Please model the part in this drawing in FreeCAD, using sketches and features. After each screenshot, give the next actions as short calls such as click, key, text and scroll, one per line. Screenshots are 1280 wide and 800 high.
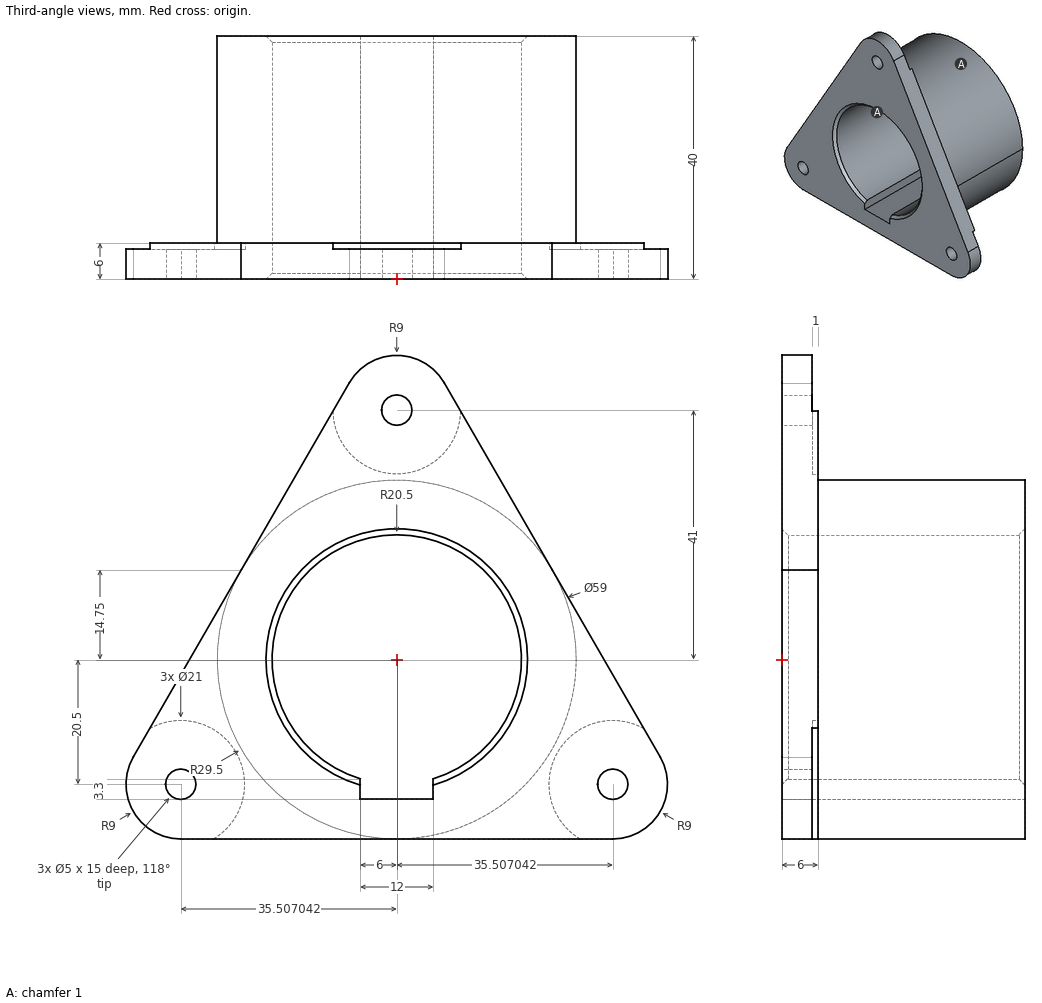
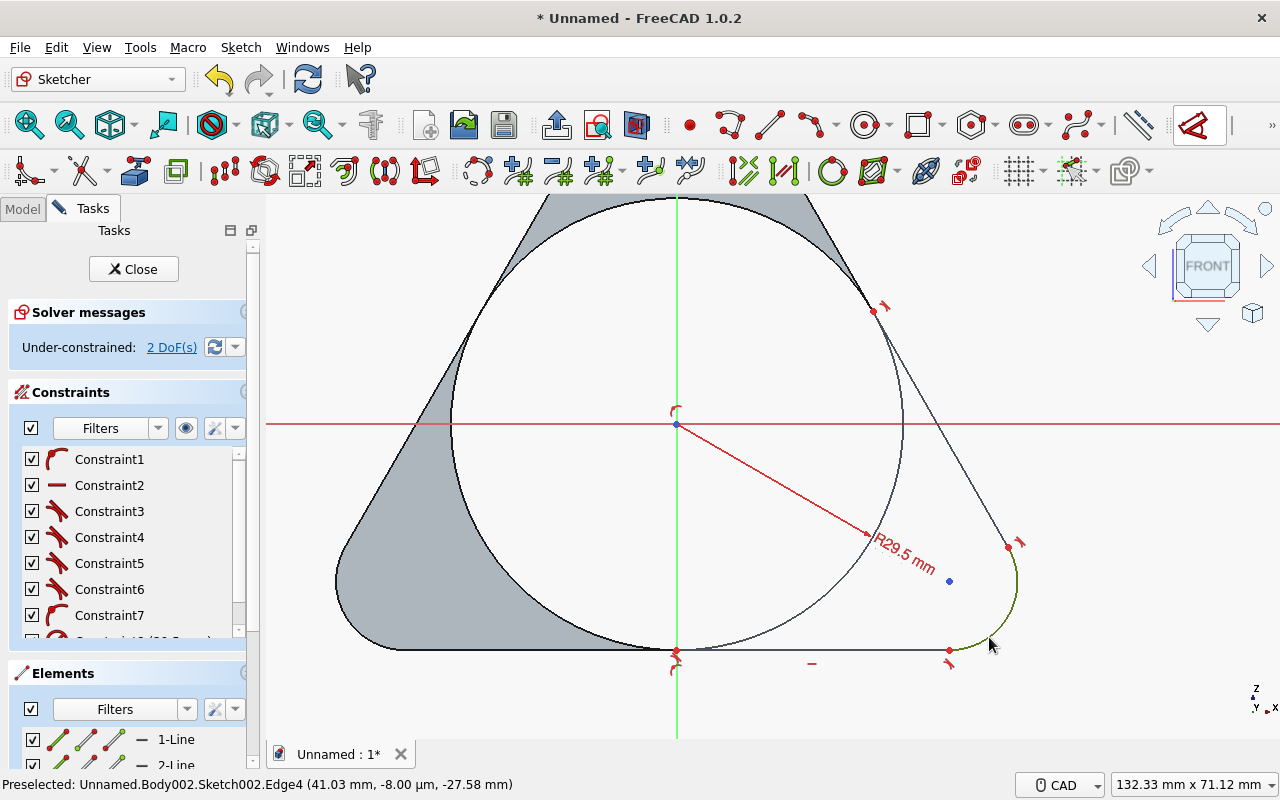
key(k)
key(r)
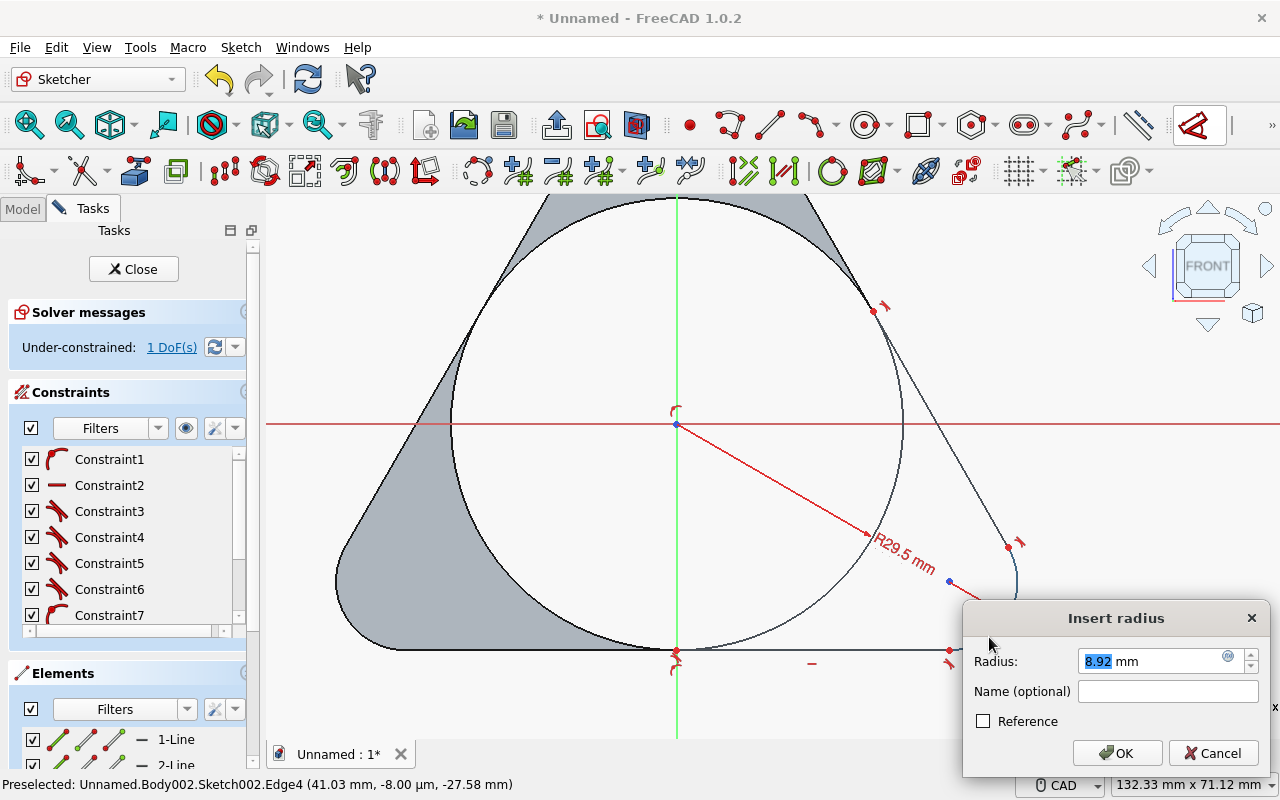
text(9)
key(Return)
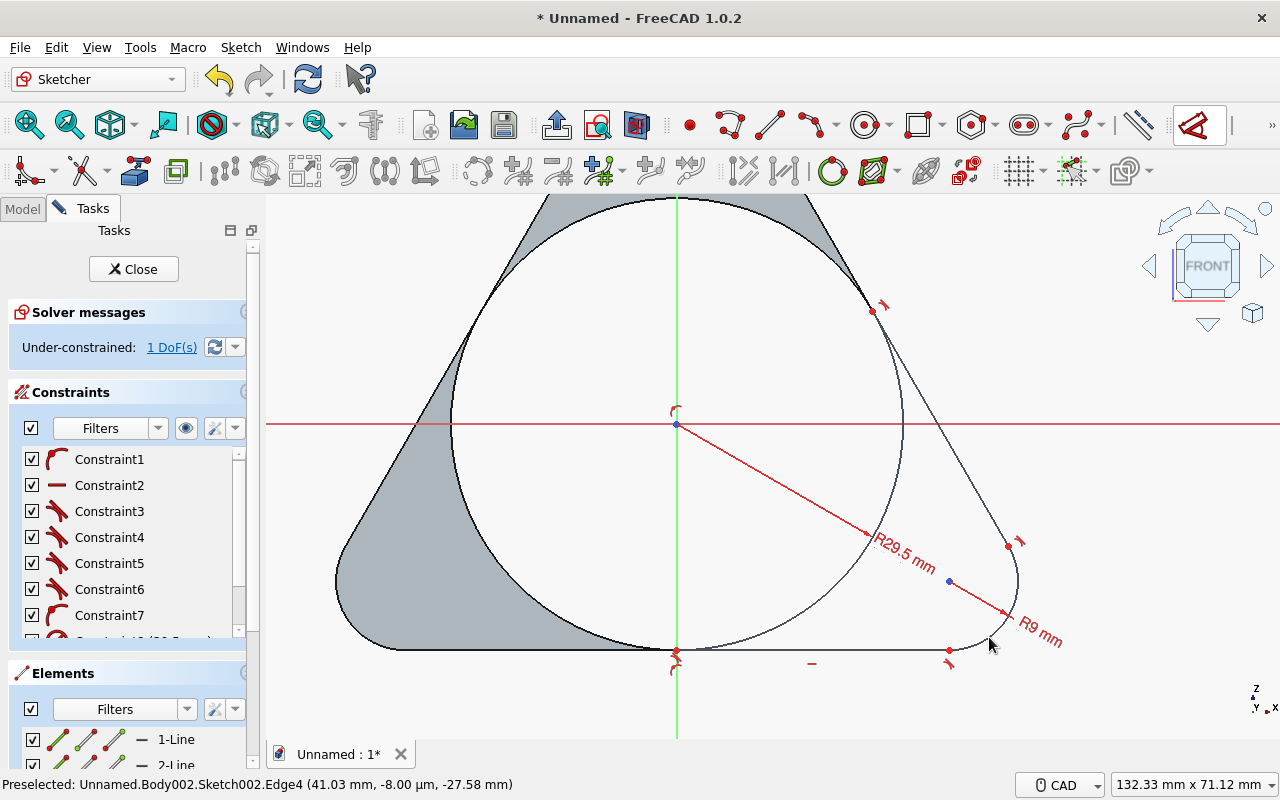
click(873, 311)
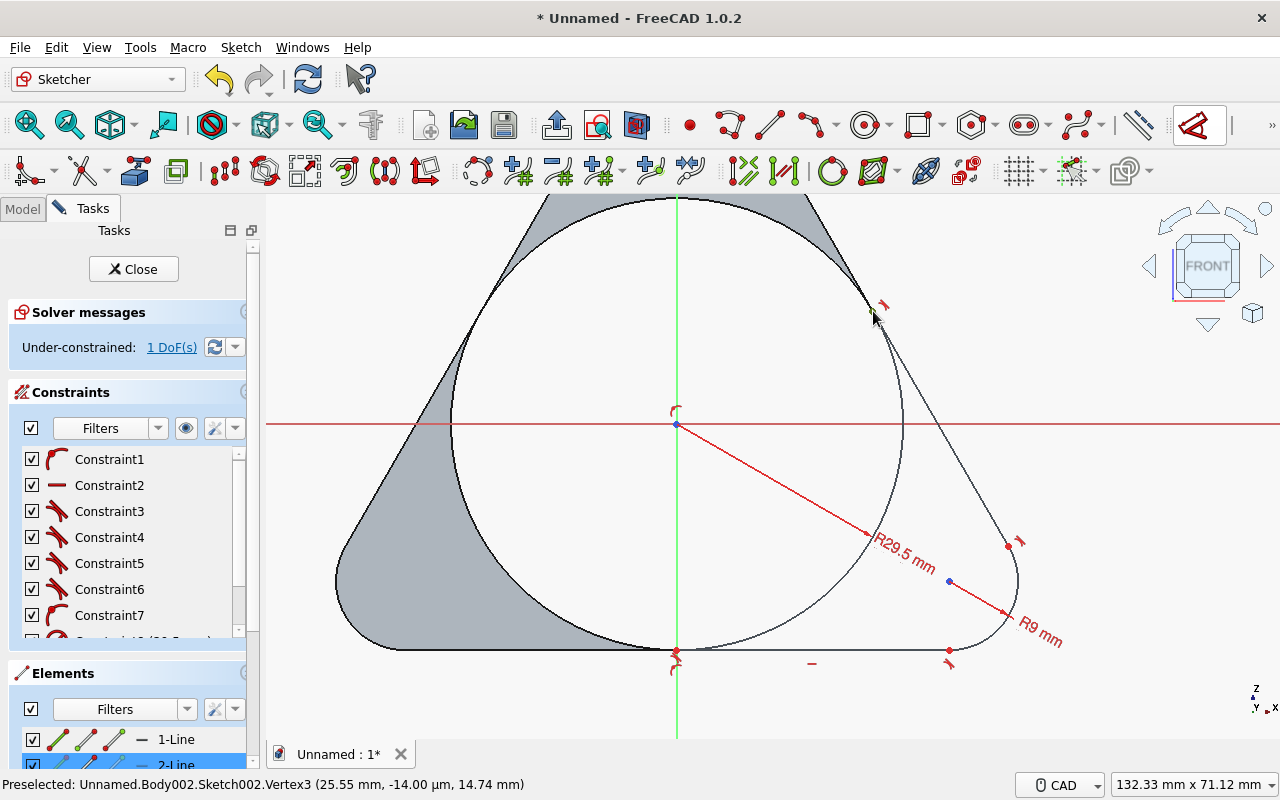
click(1220, 126)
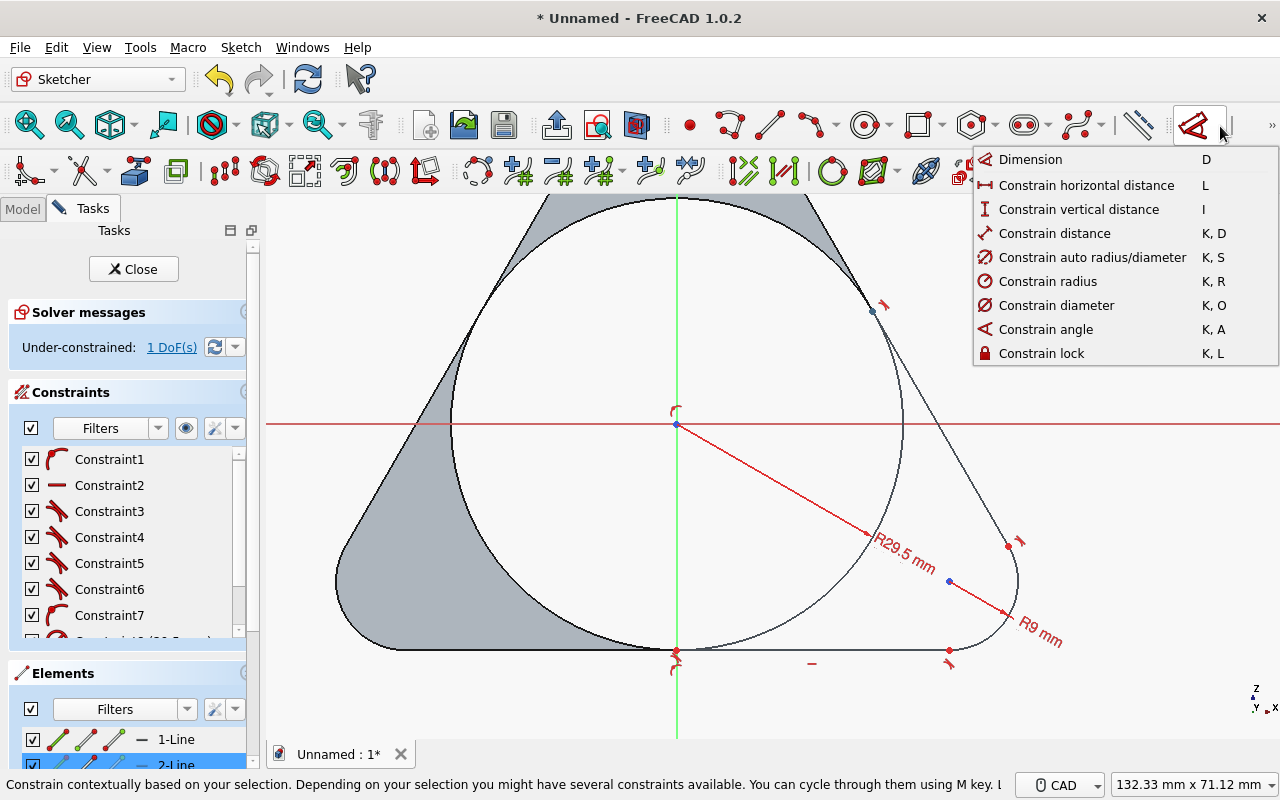
click(1126, 209)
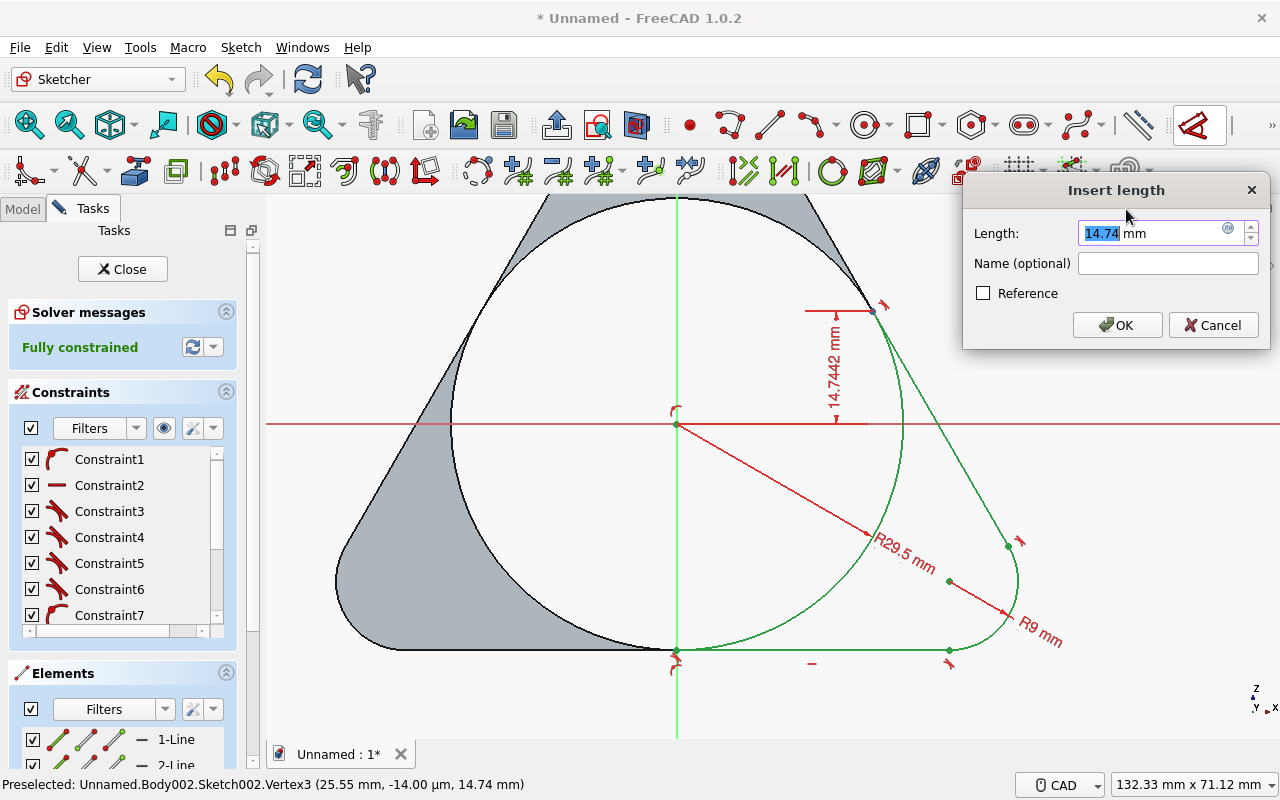
text(14.75)
key(Return)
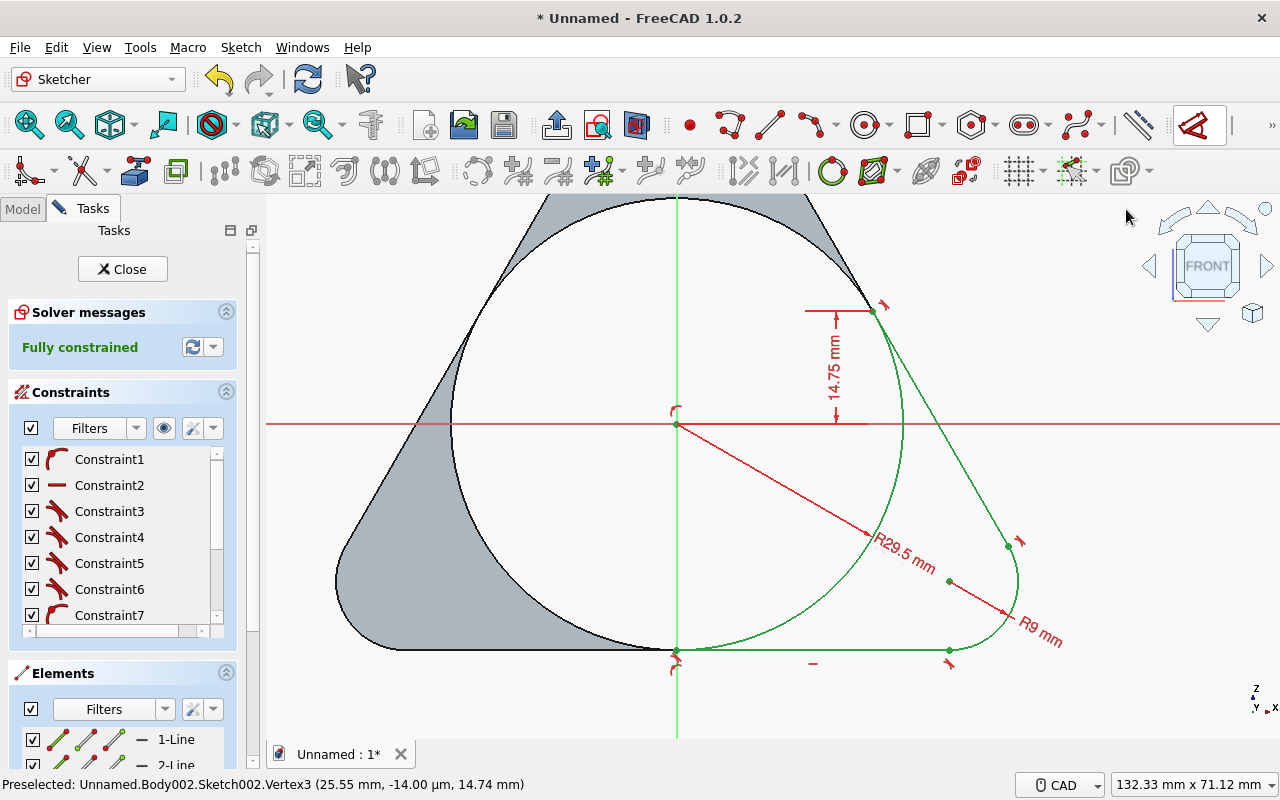
click(123, 269)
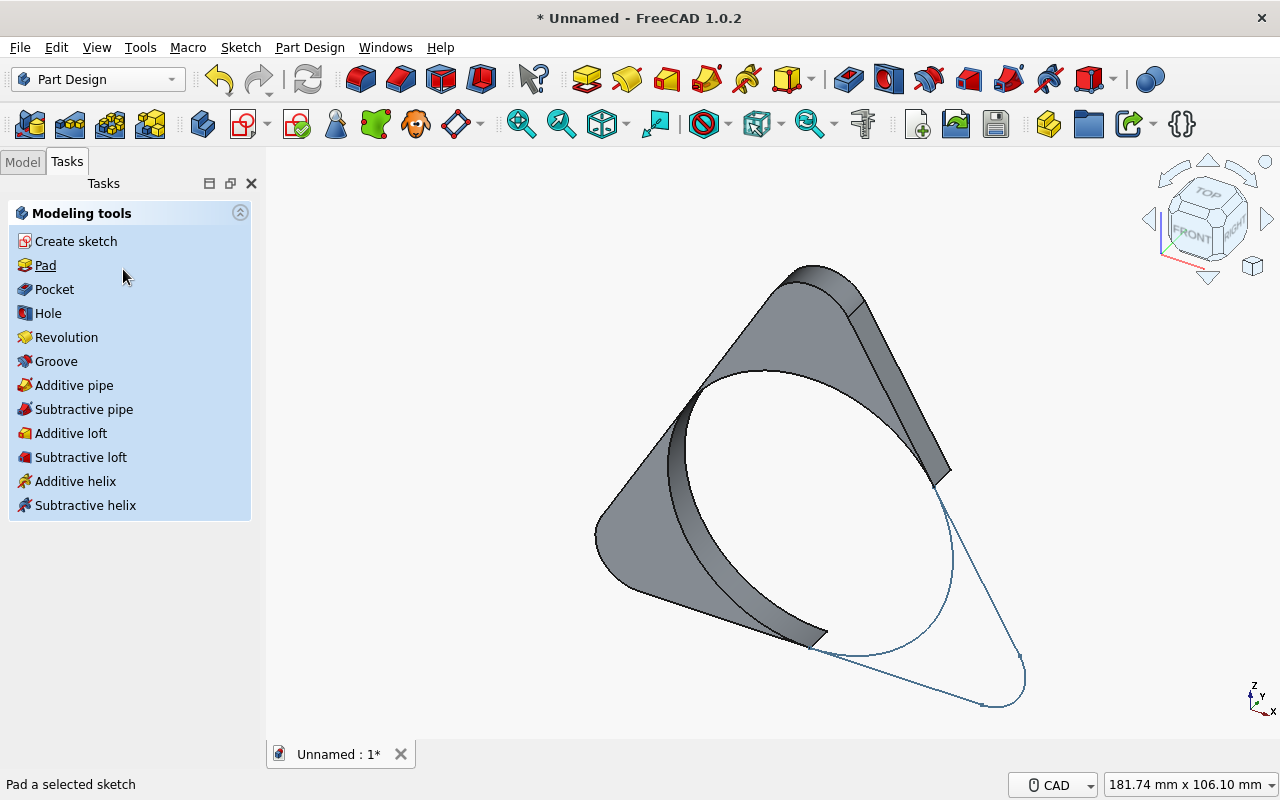
click(588, 80)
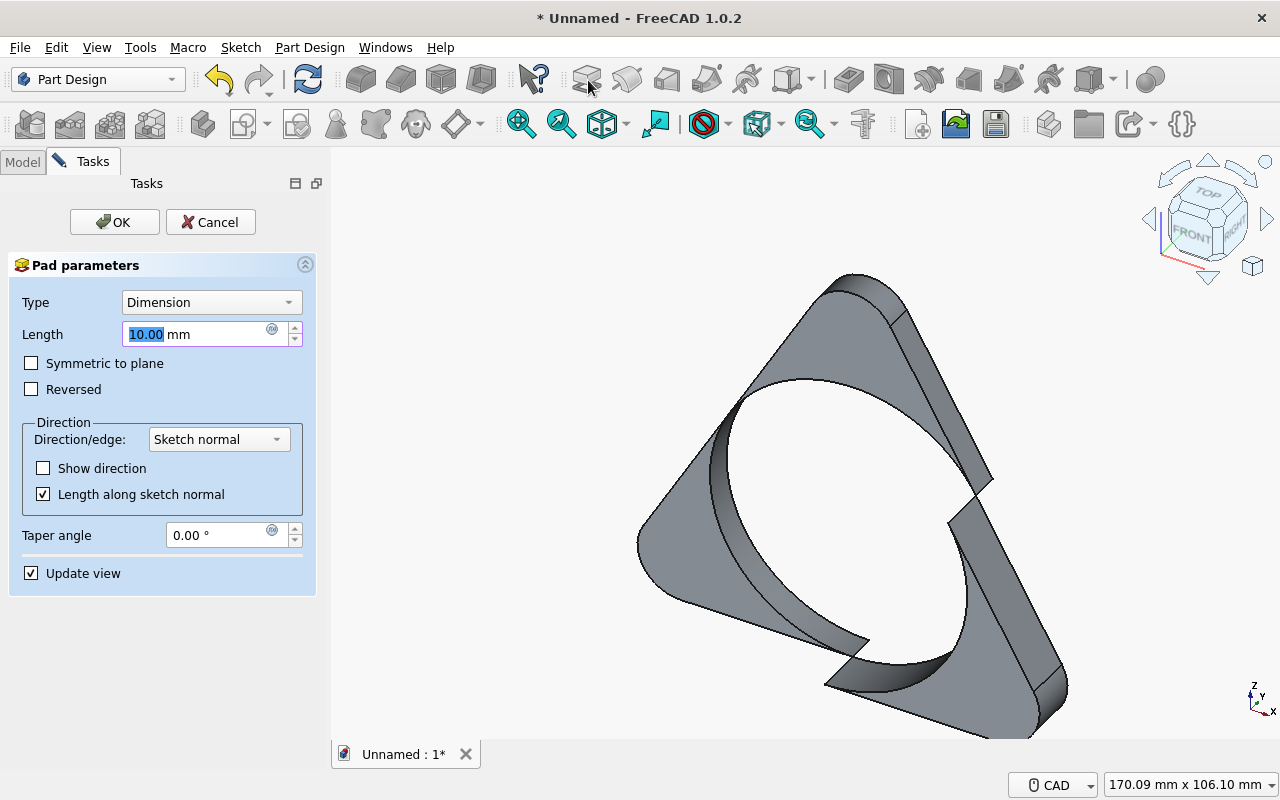
text(6)
key(Tab)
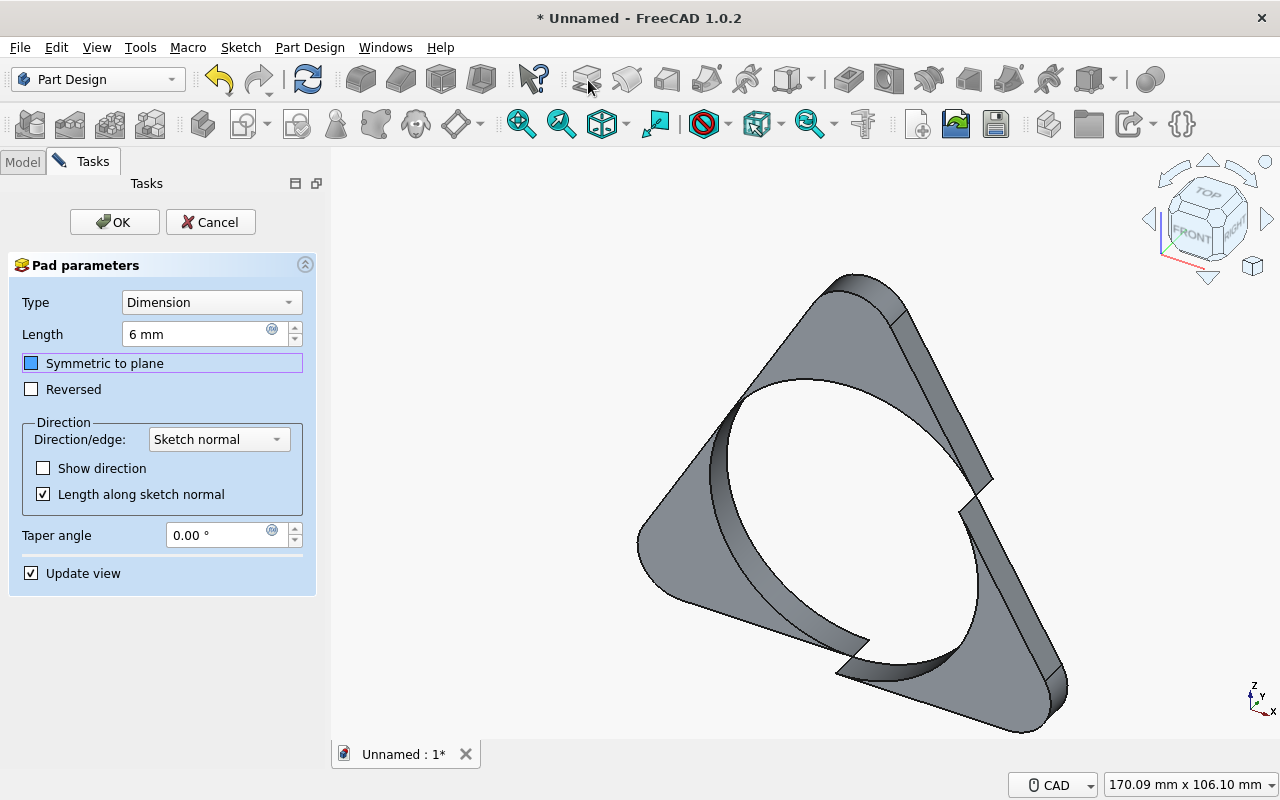
click(30, 389)